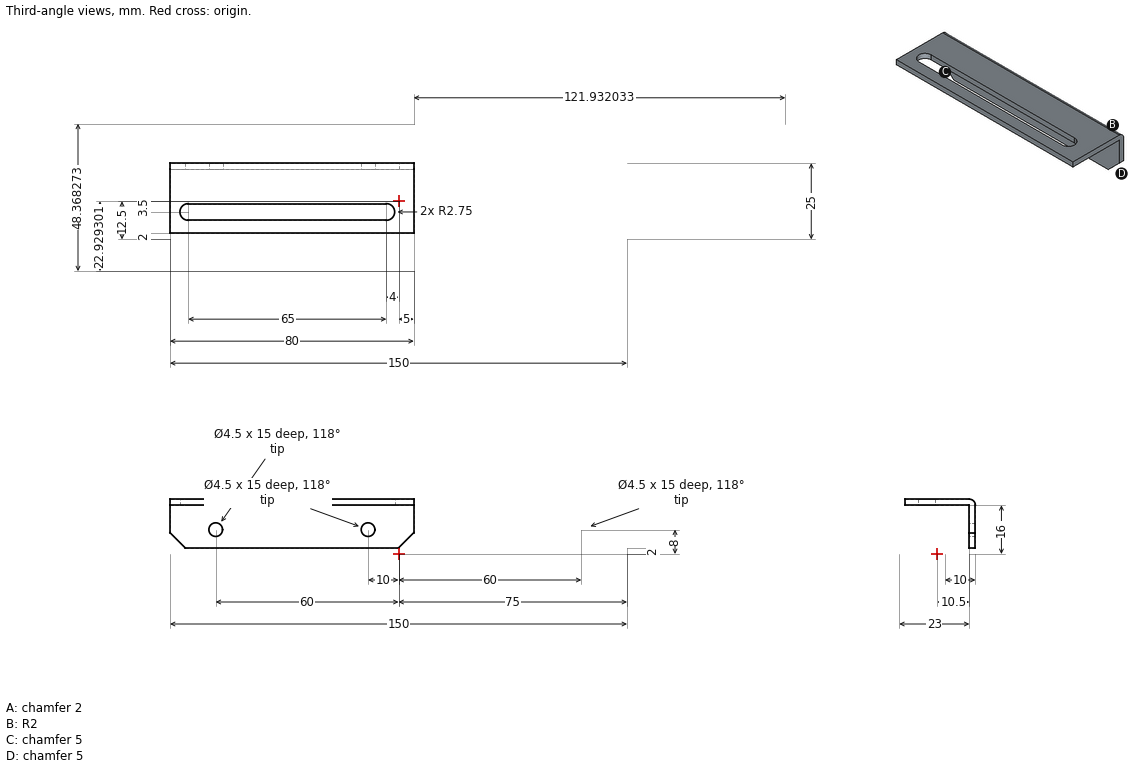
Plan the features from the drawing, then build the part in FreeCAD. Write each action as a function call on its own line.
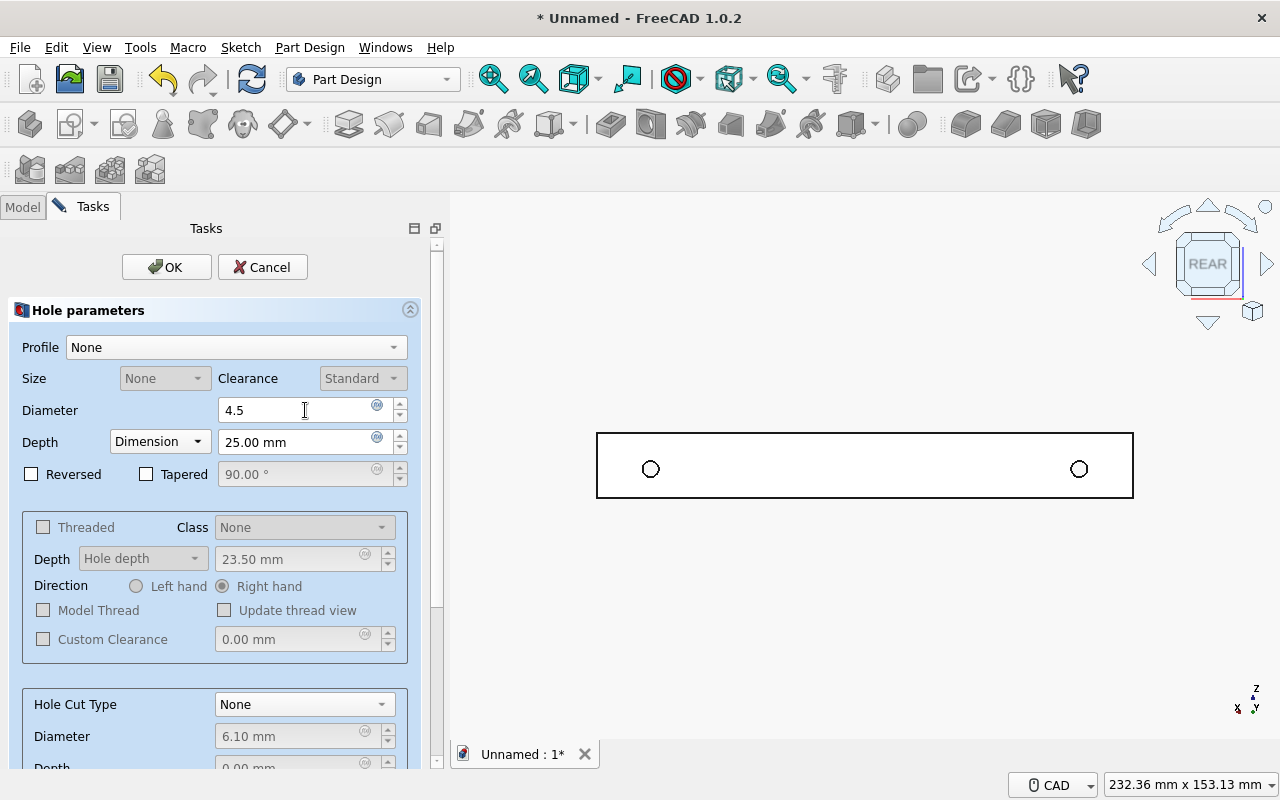
triple_click(305, 442)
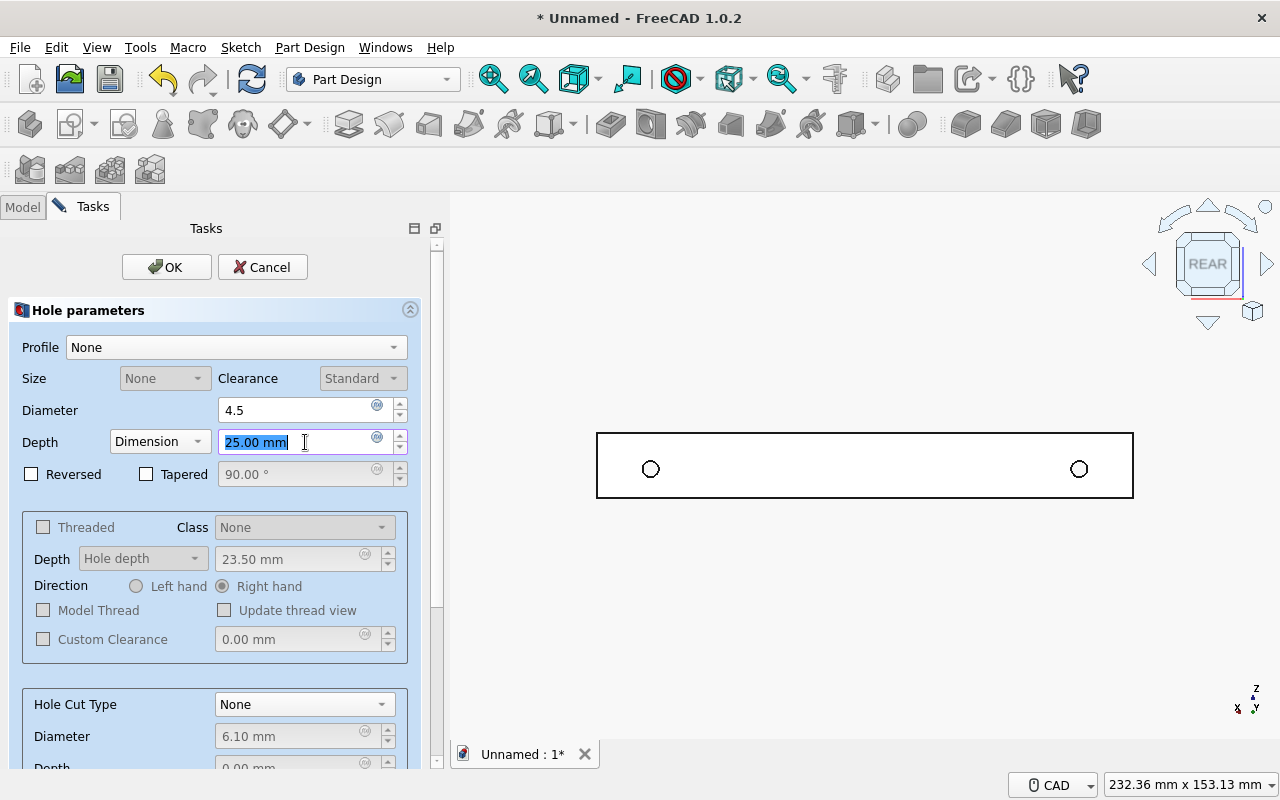
text(15)
key(Tab)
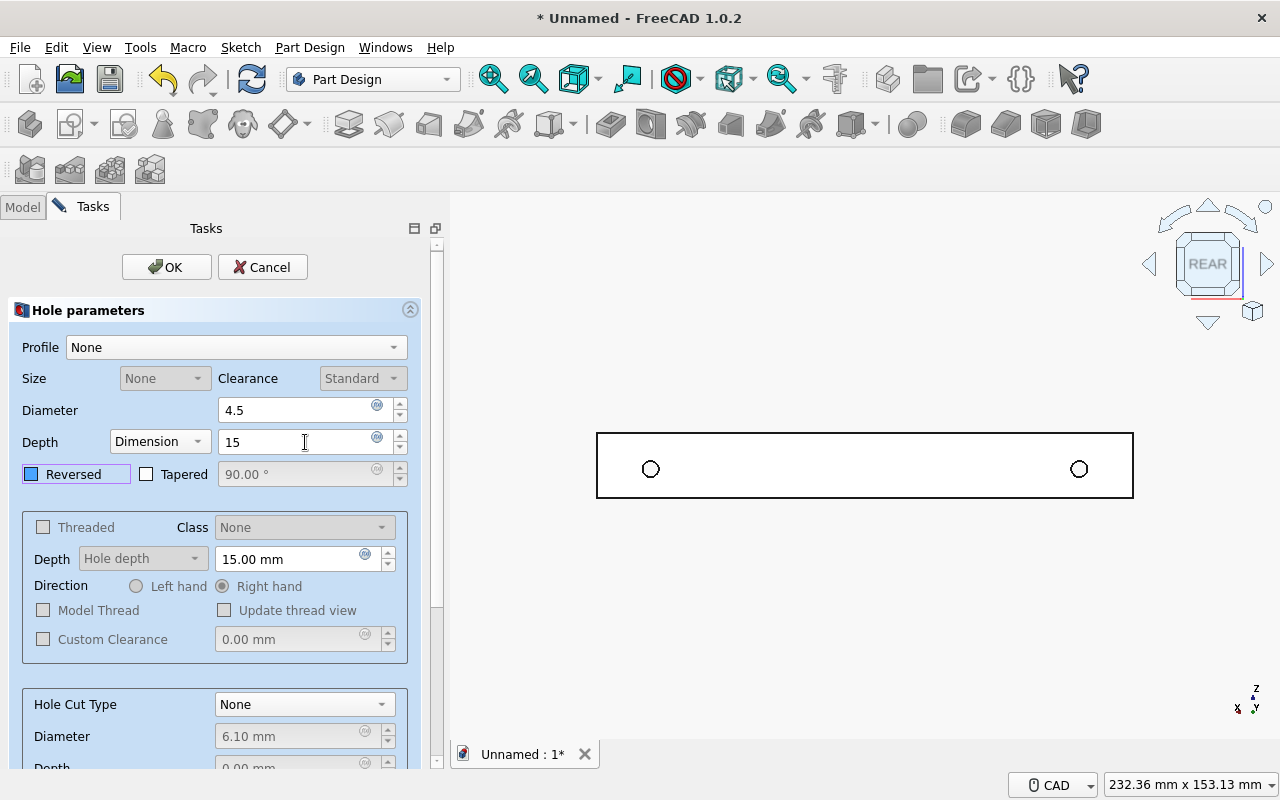
click(167, 267)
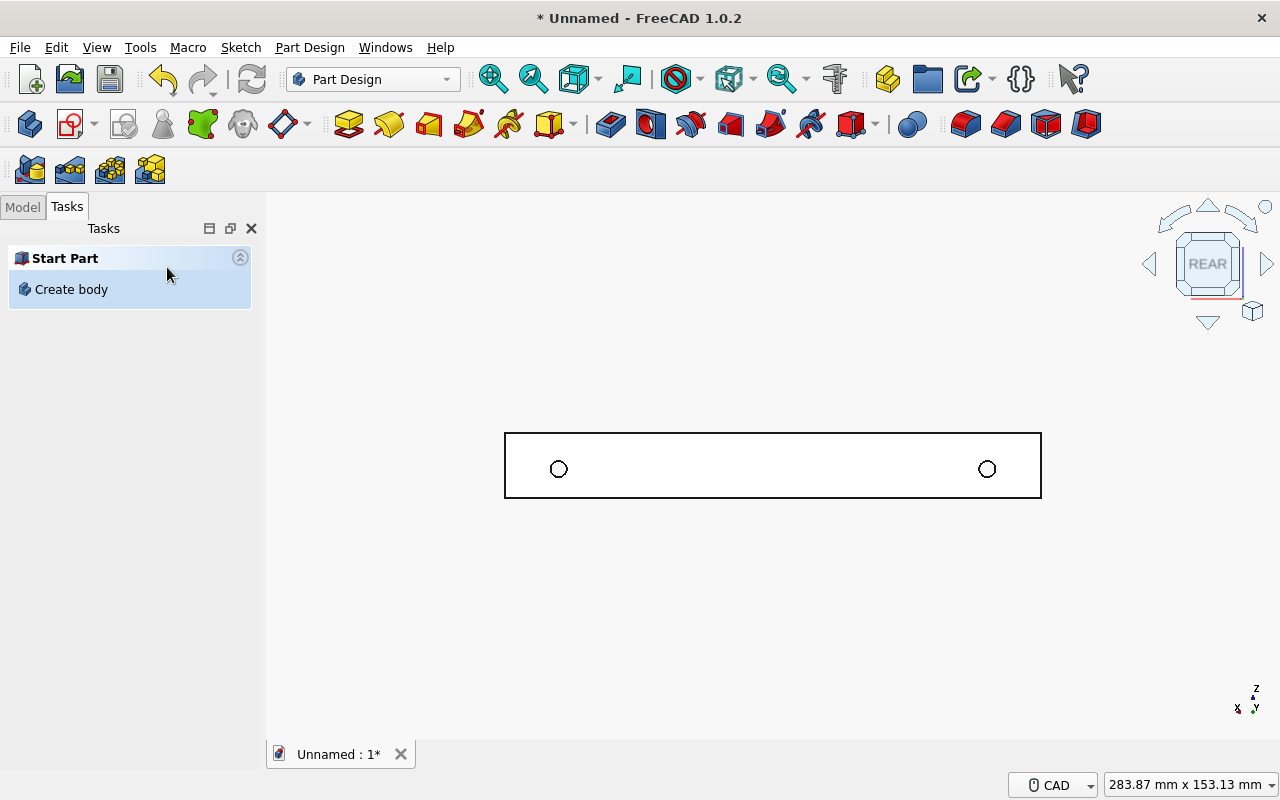
click(620, 464)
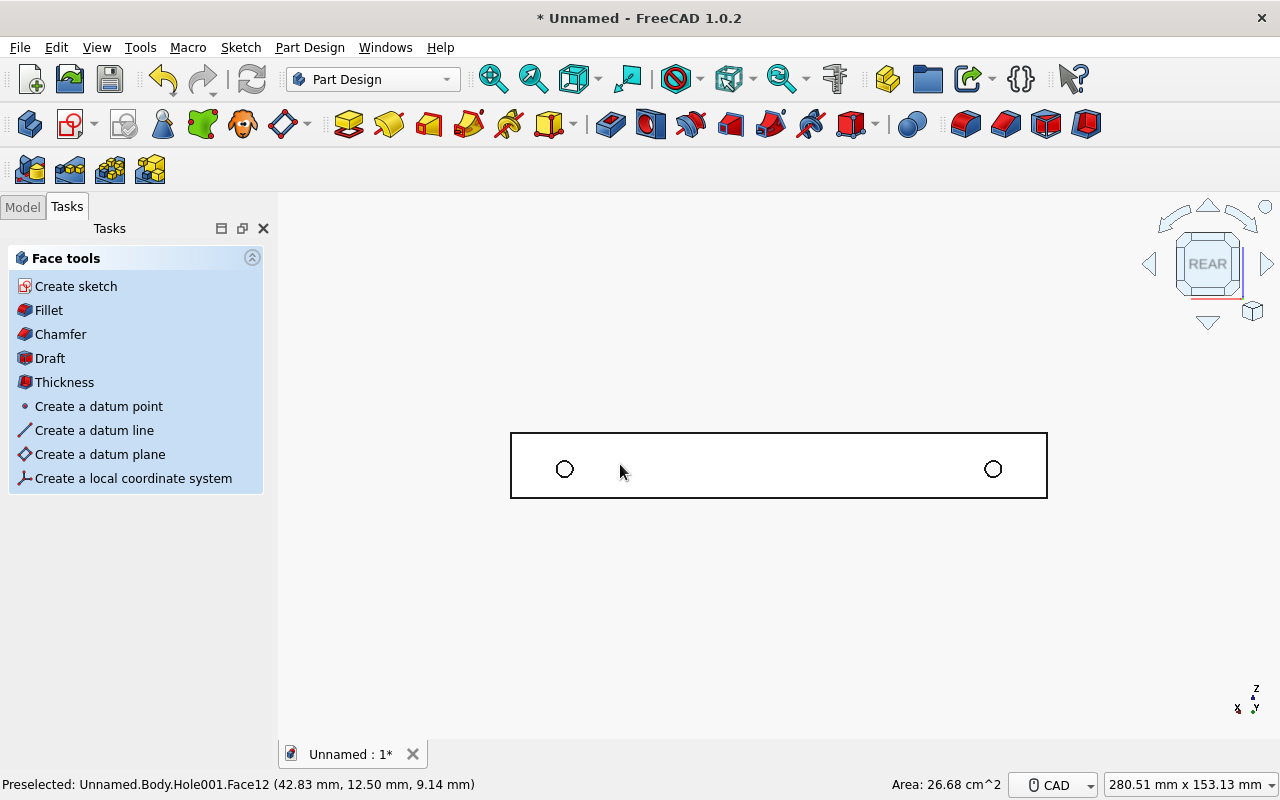
click(70, 124)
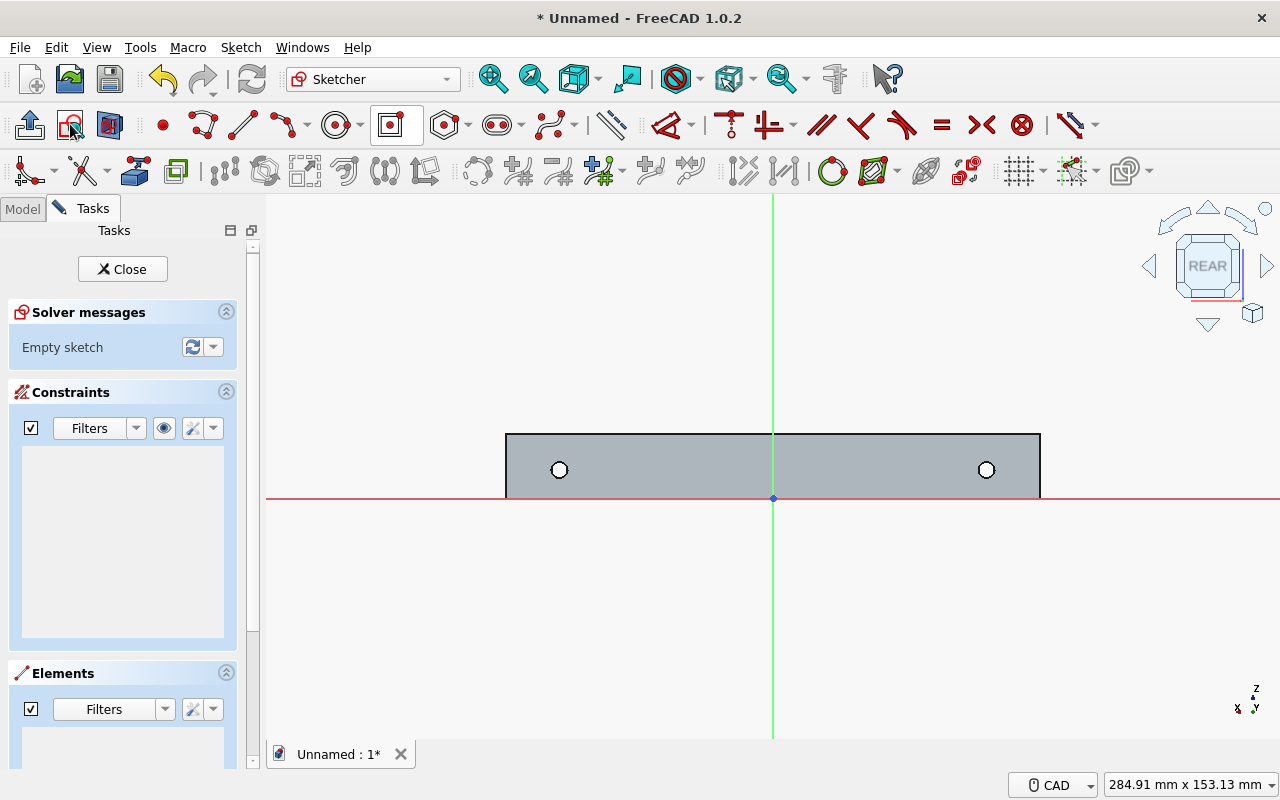
scroll(814, 470, up, 15)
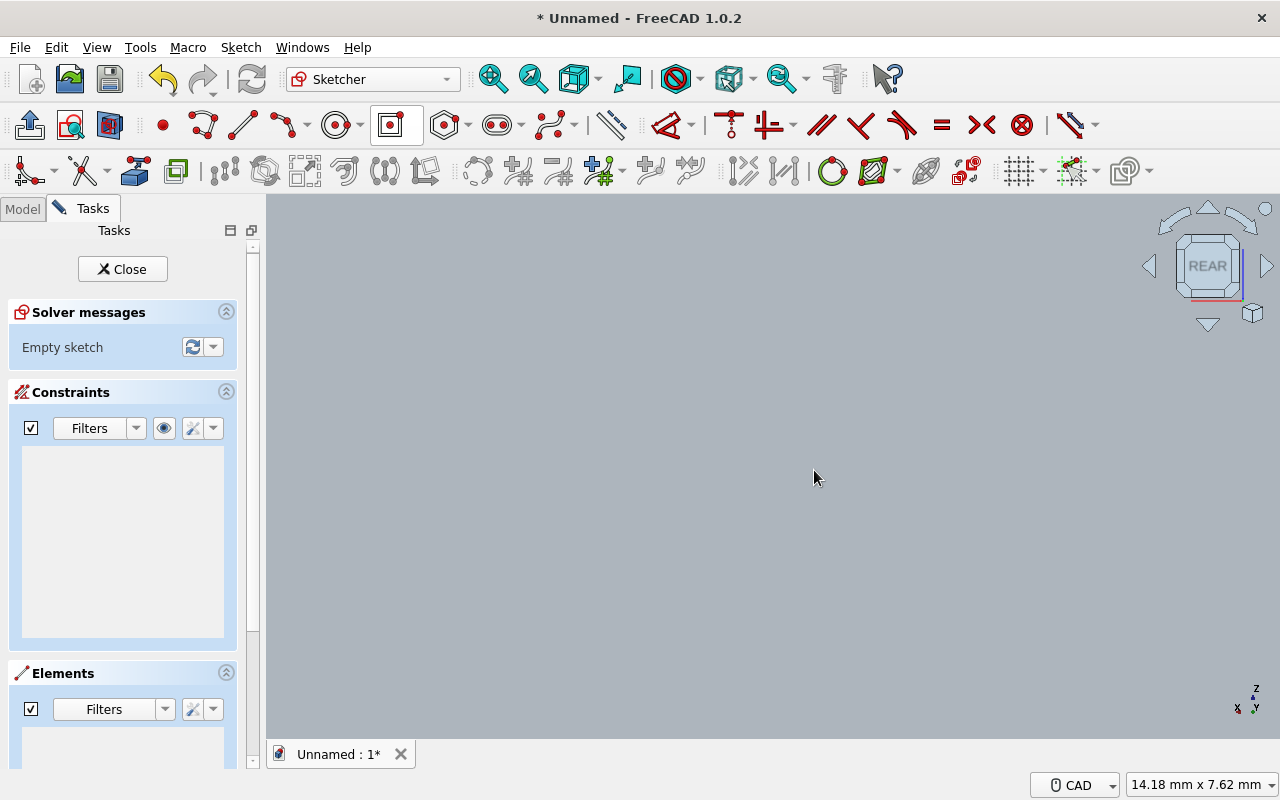
click(336, 126)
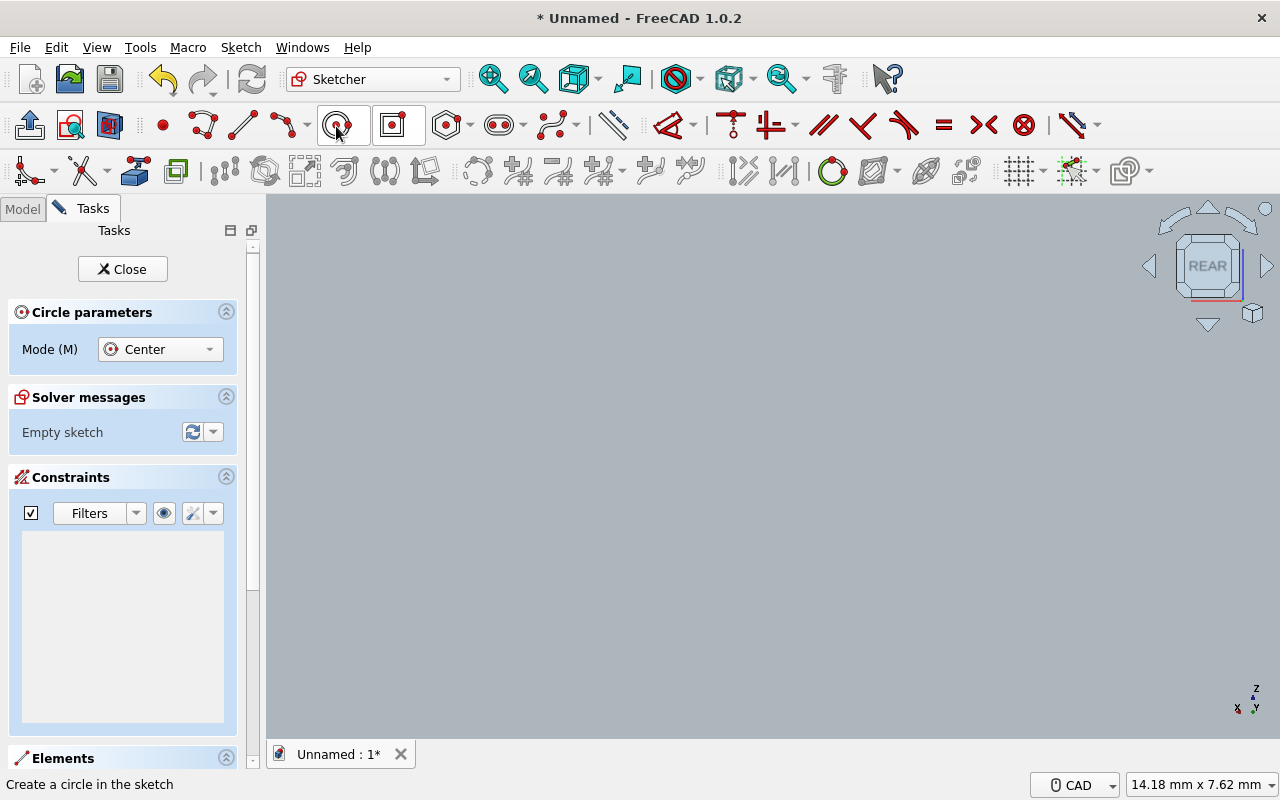
click(695, 462)
click(809, 348)
key(Escape)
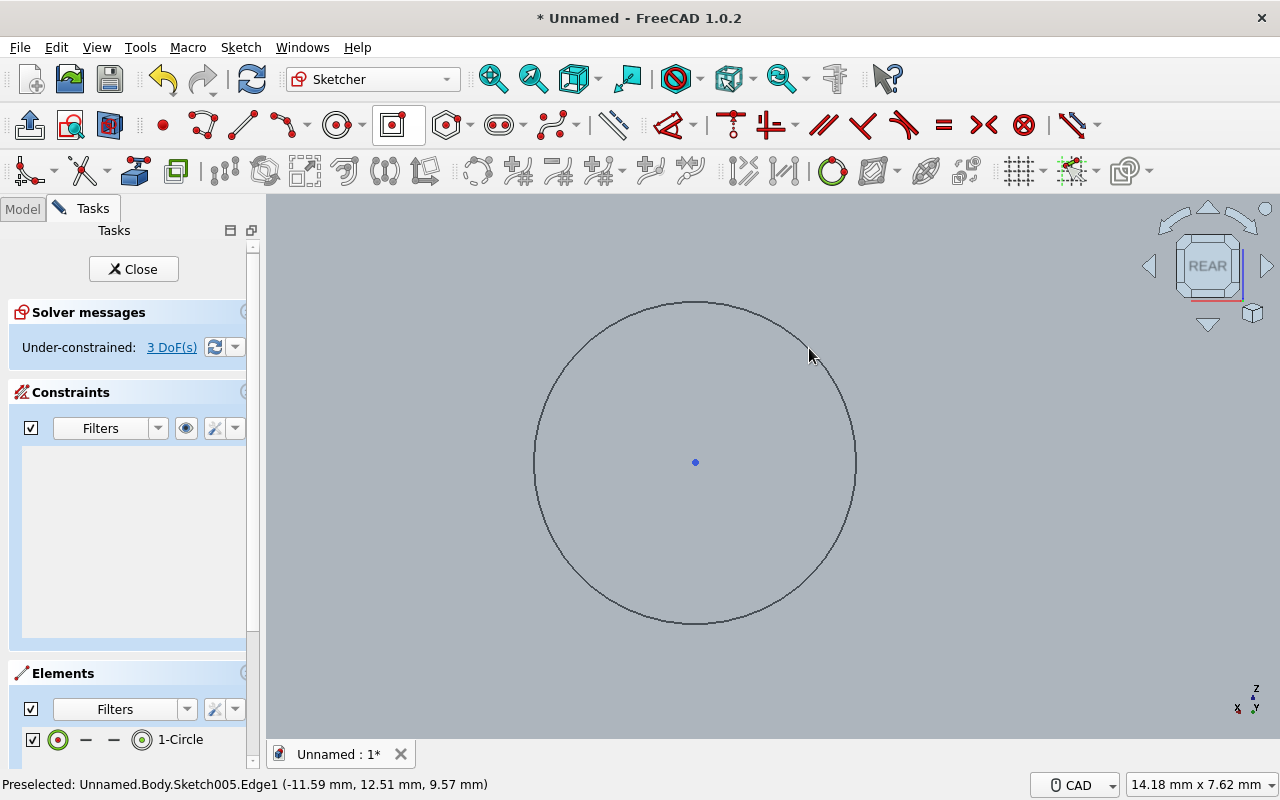
click(668, 126)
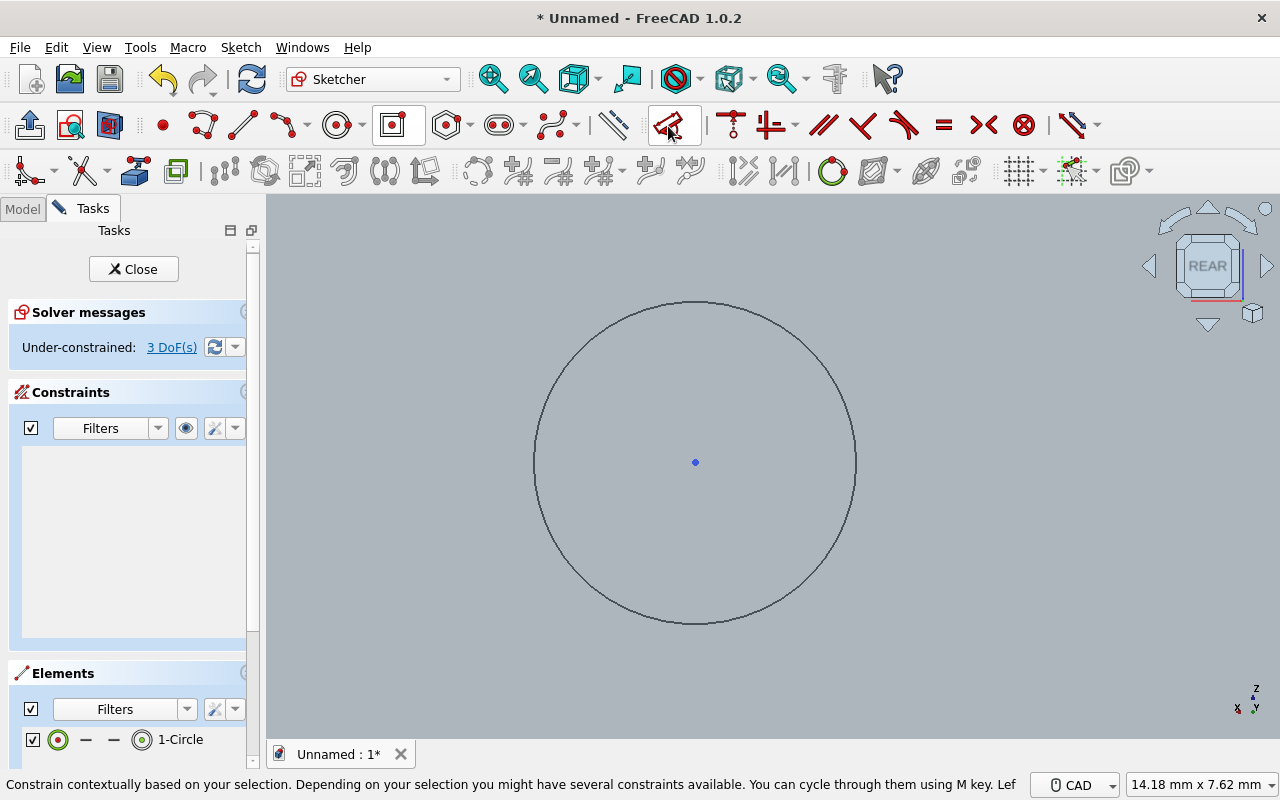
click(809, 349)
click(832, 326)